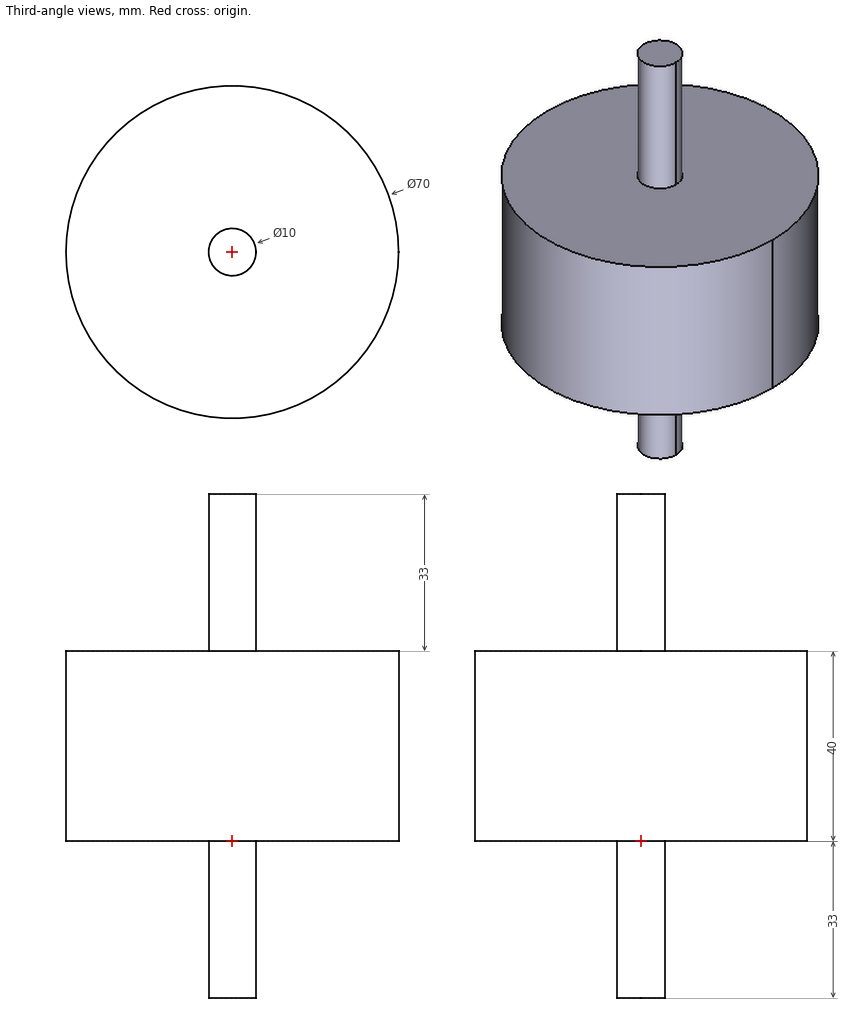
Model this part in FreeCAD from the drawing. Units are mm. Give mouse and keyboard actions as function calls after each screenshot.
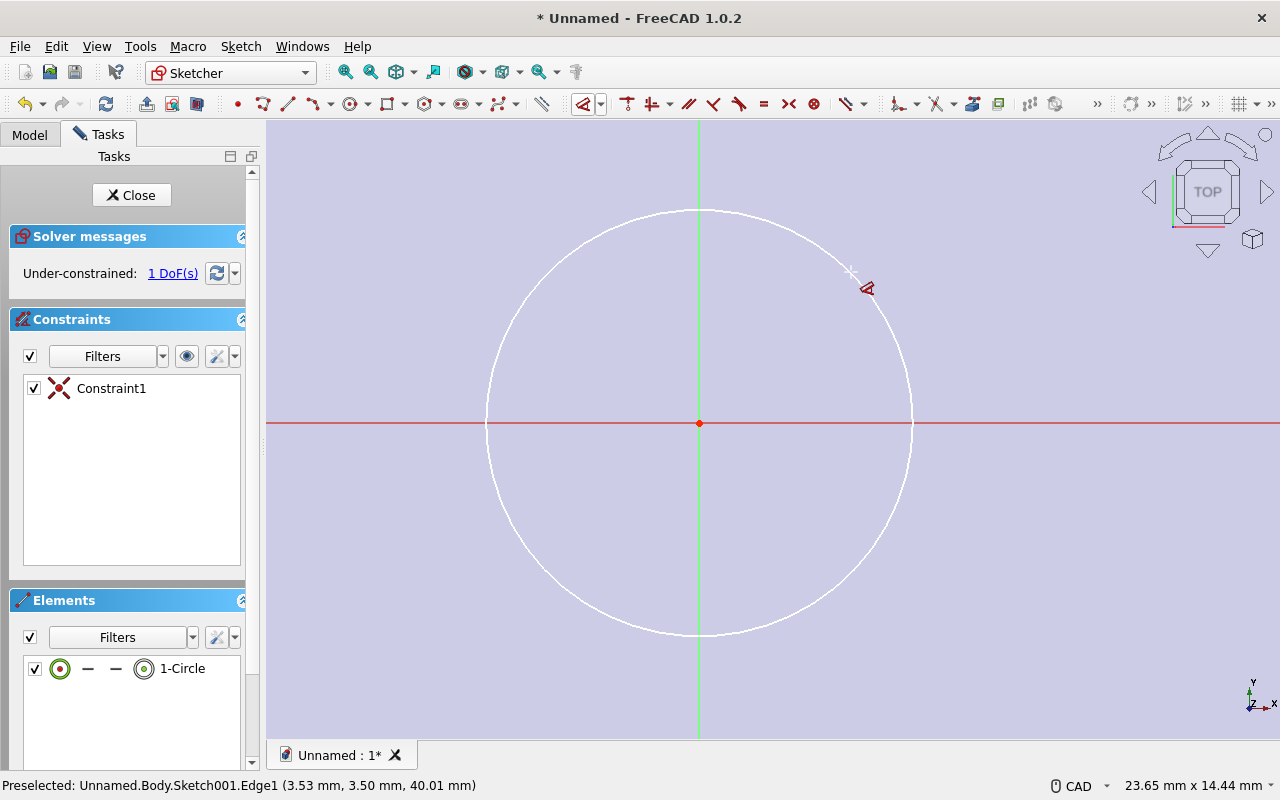
click(850, 272)
click(873, 249)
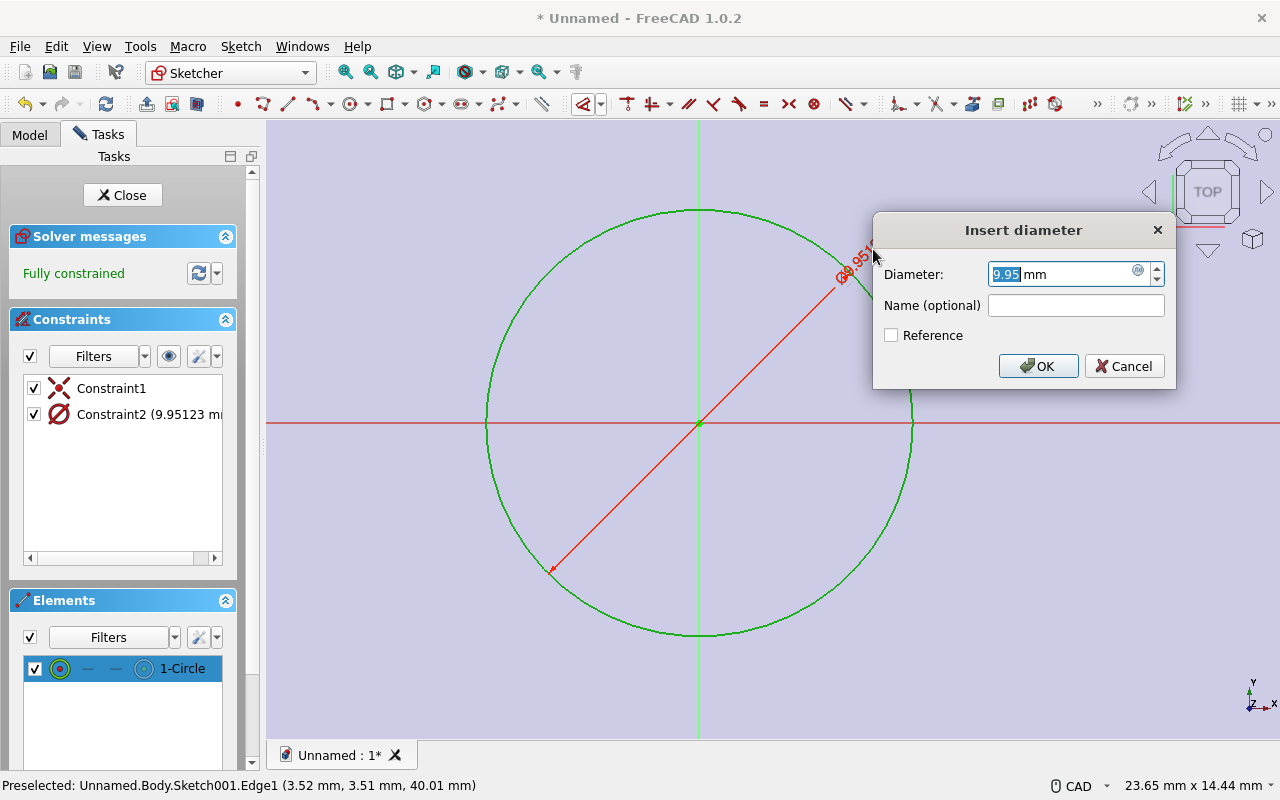
text(10)
key(Return)
key(Escape)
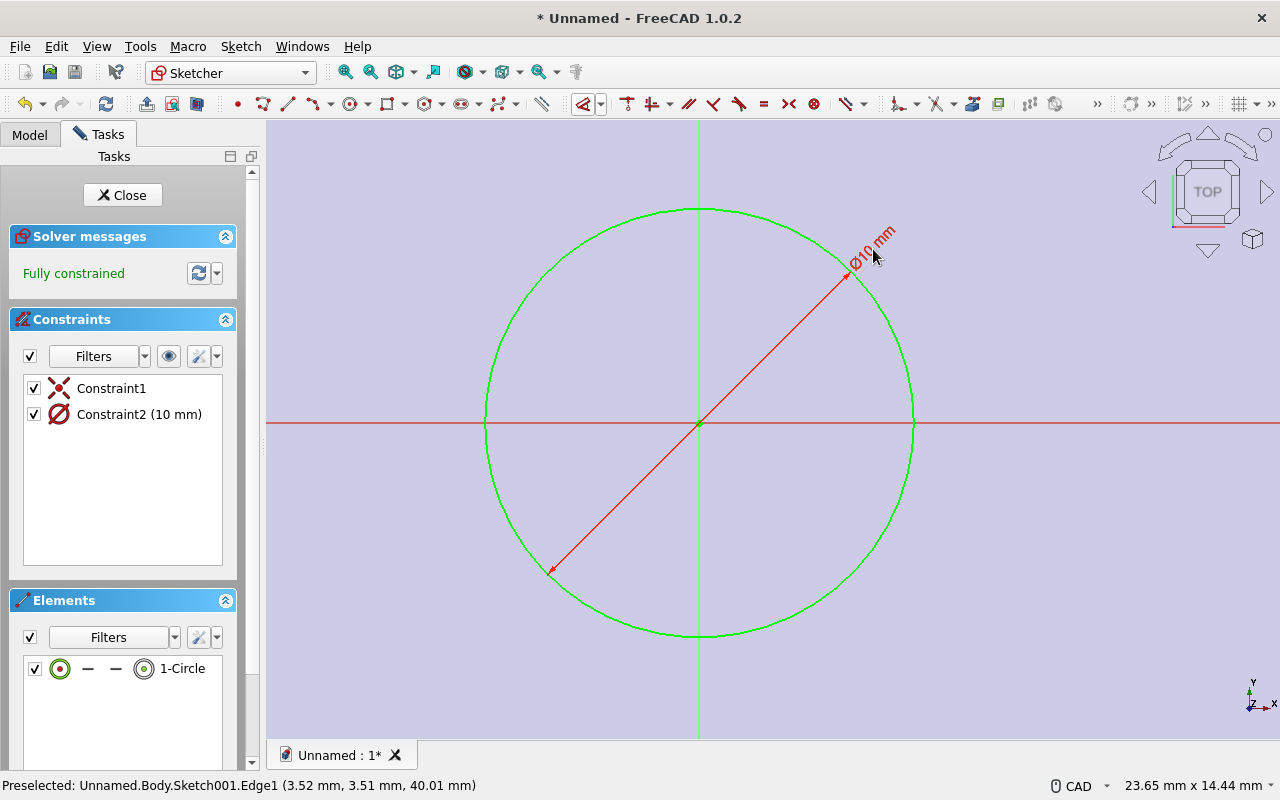
click(123, 195)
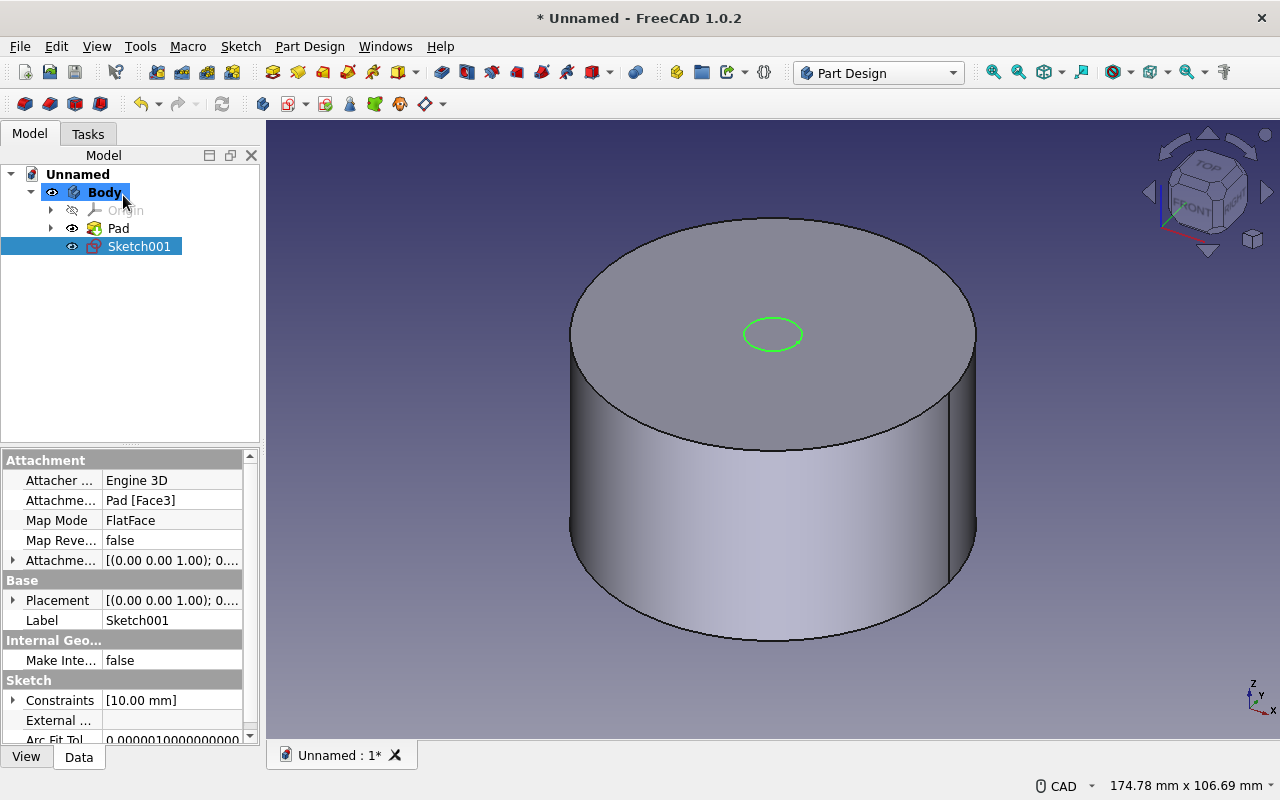
click(273, 72)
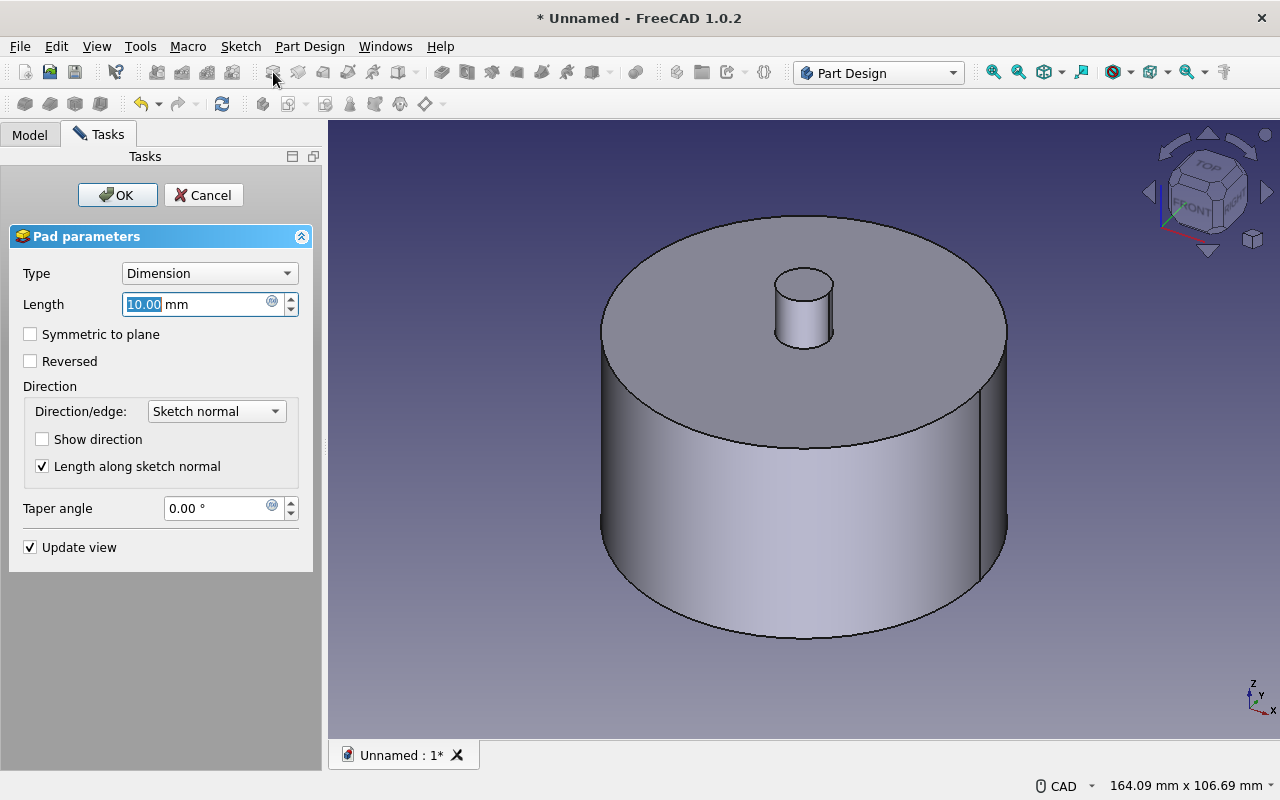
text(33)
key(Tab)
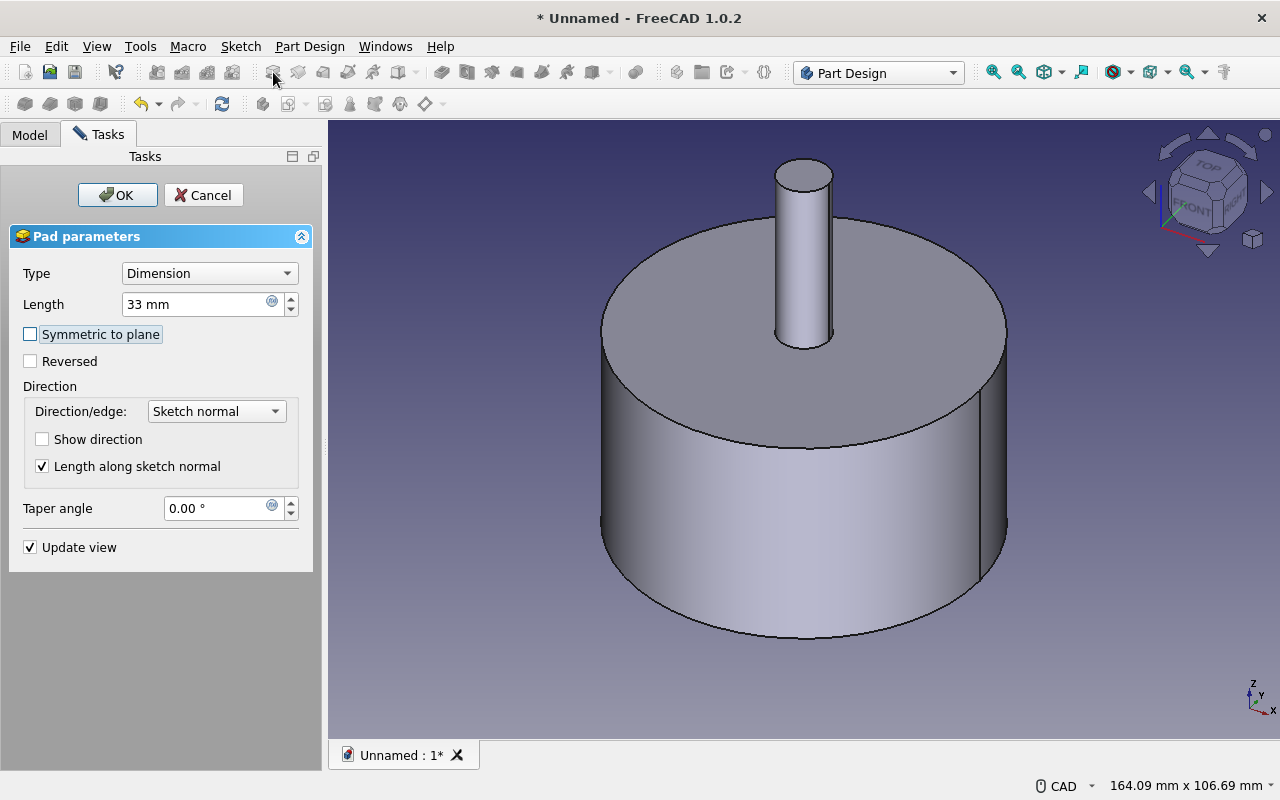
click(118, 195)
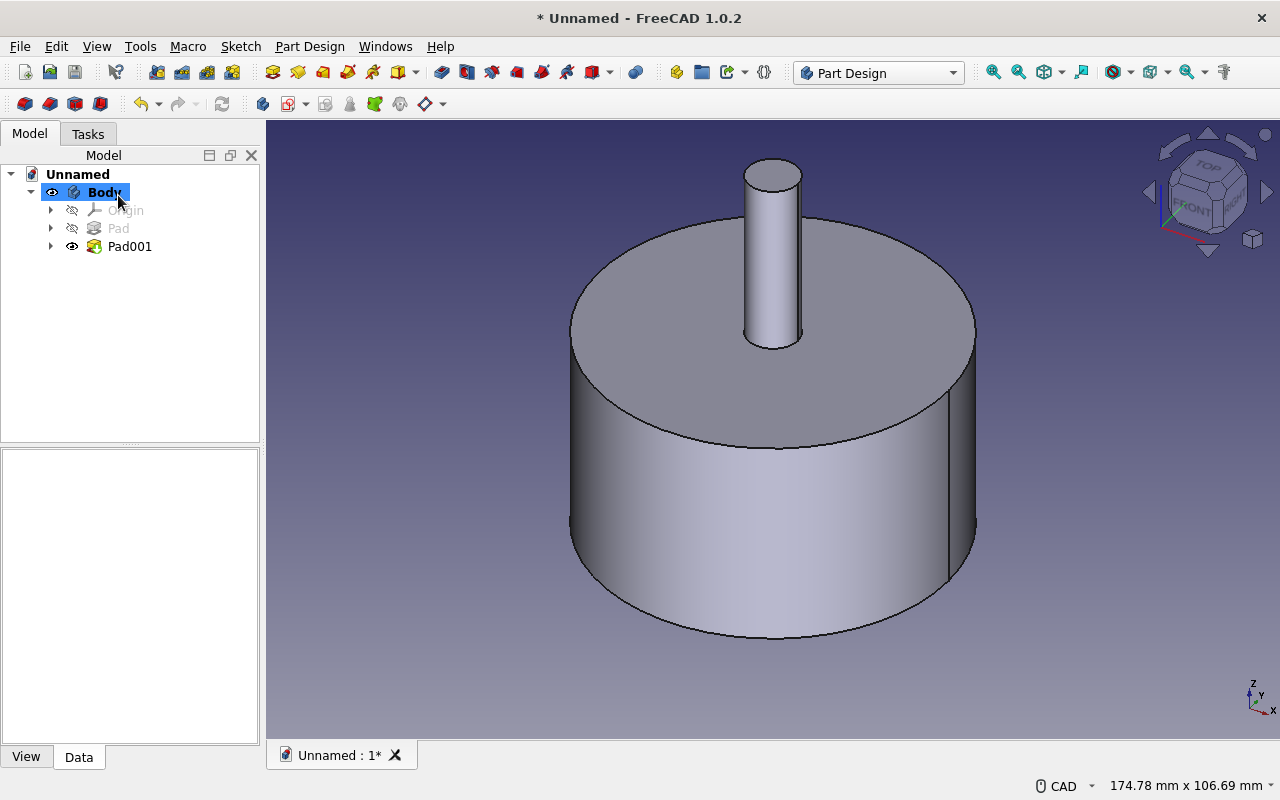
click(994, 72)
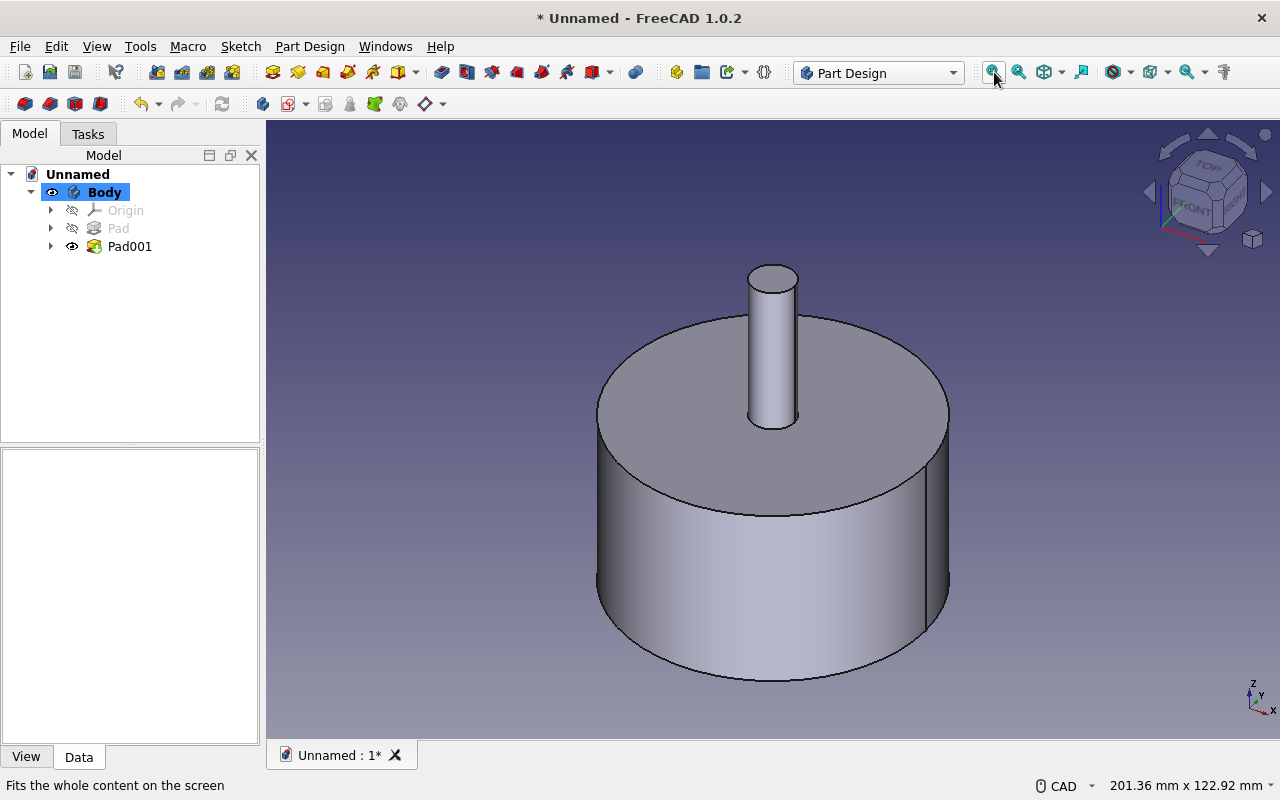
click(51, 210)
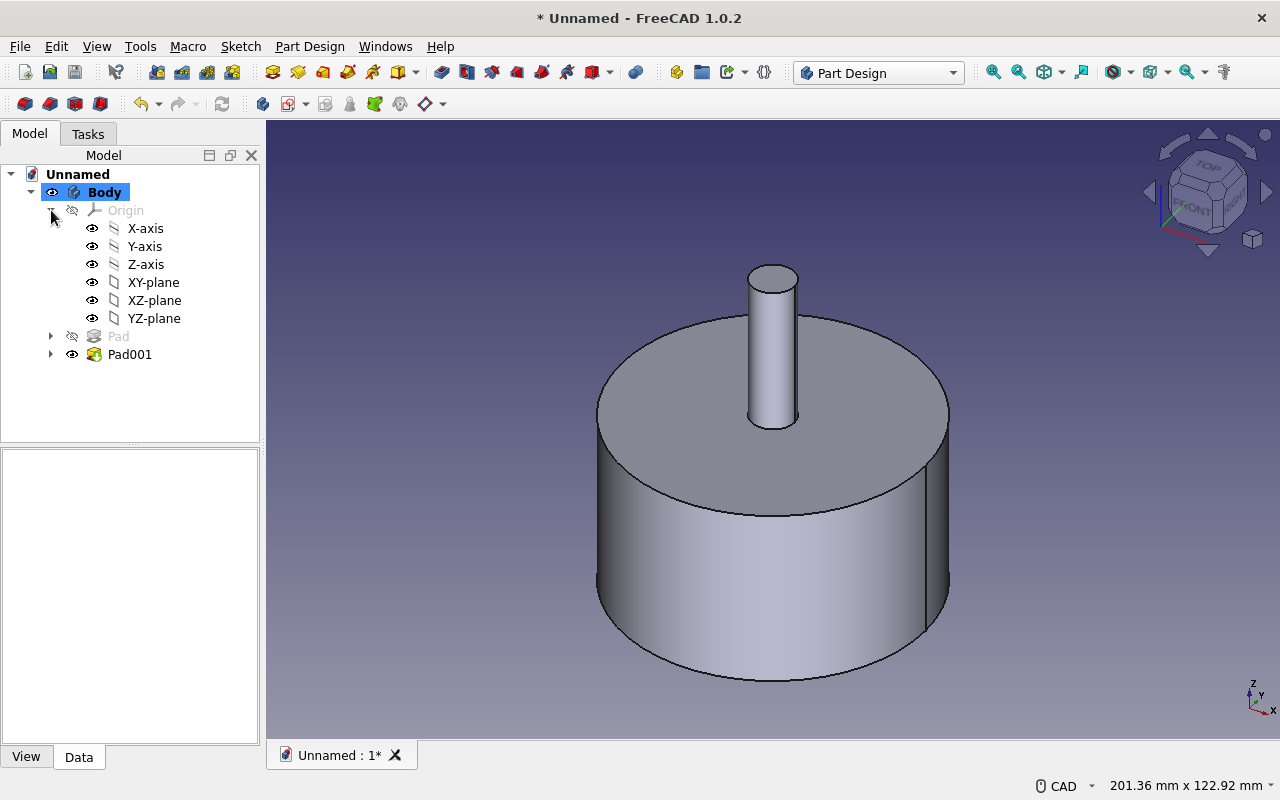
click(137, 282)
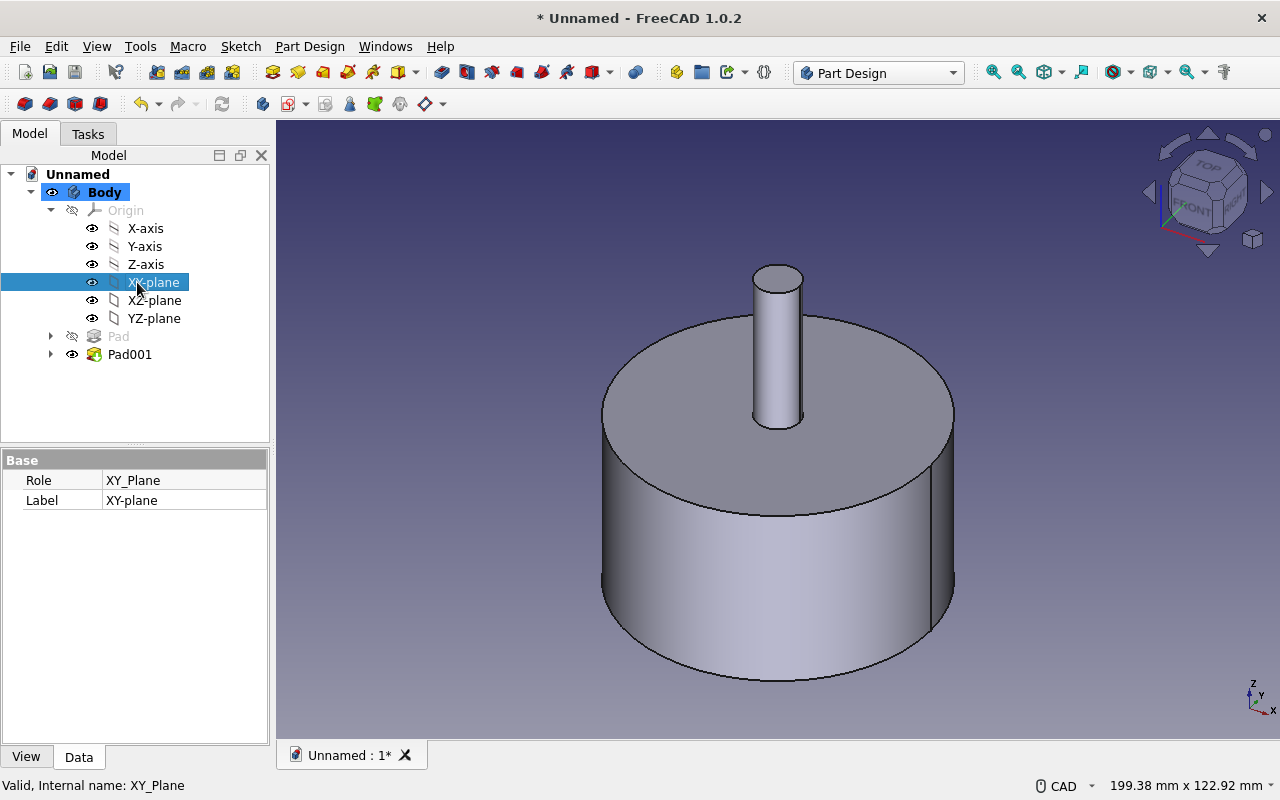
click(424, 104)